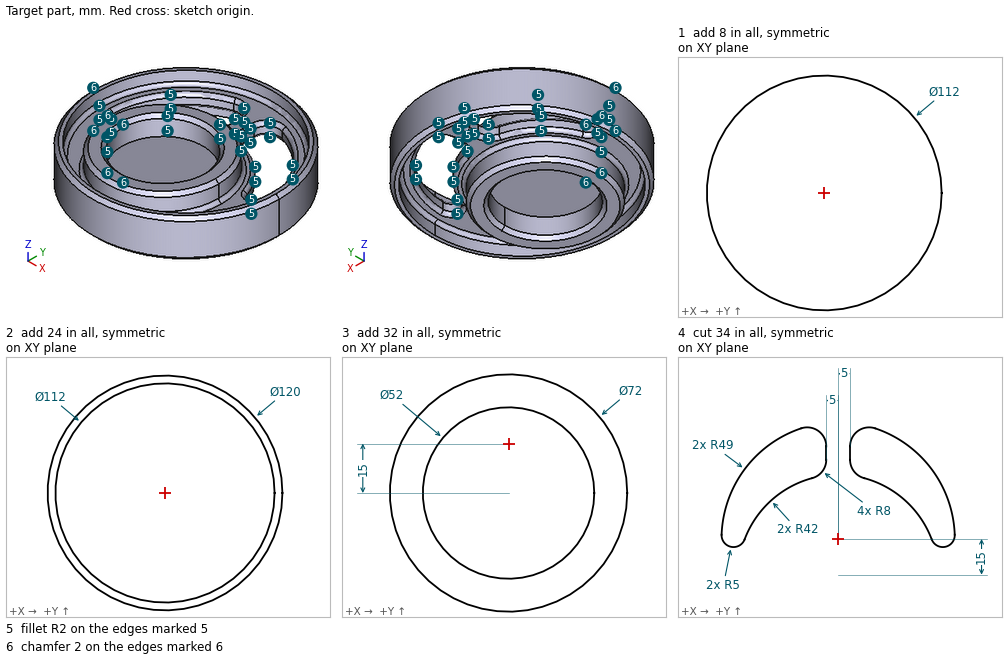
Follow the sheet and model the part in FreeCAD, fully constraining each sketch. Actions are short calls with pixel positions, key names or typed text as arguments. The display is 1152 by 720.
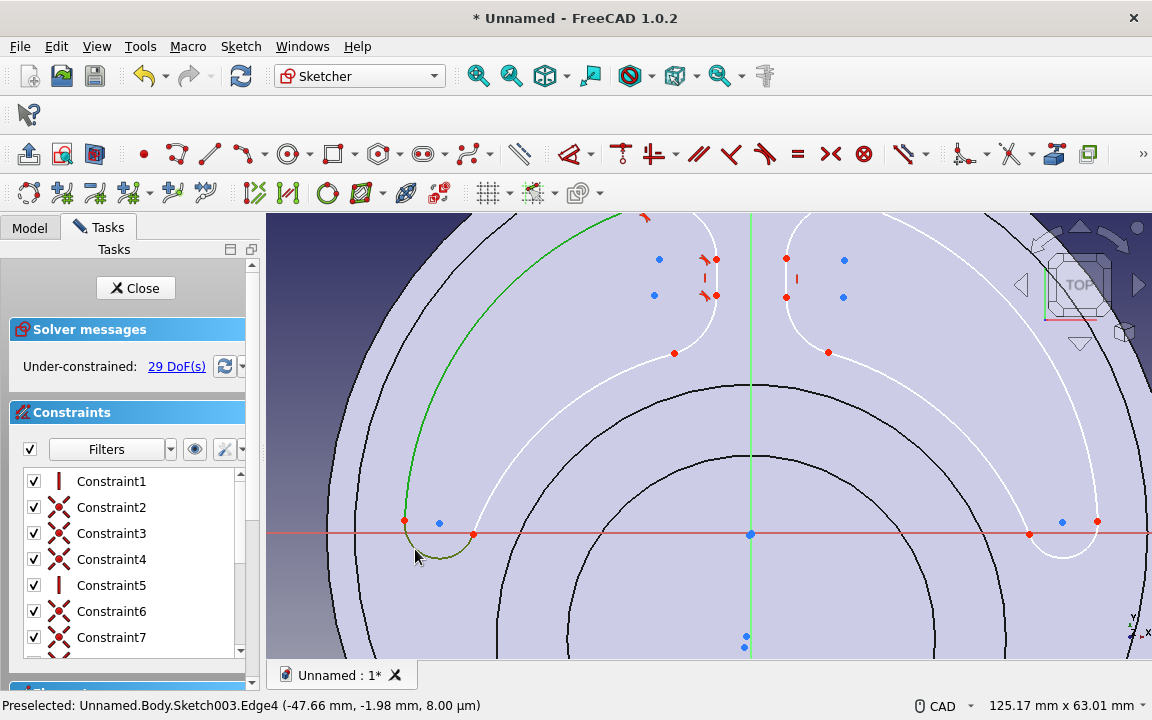
key(t)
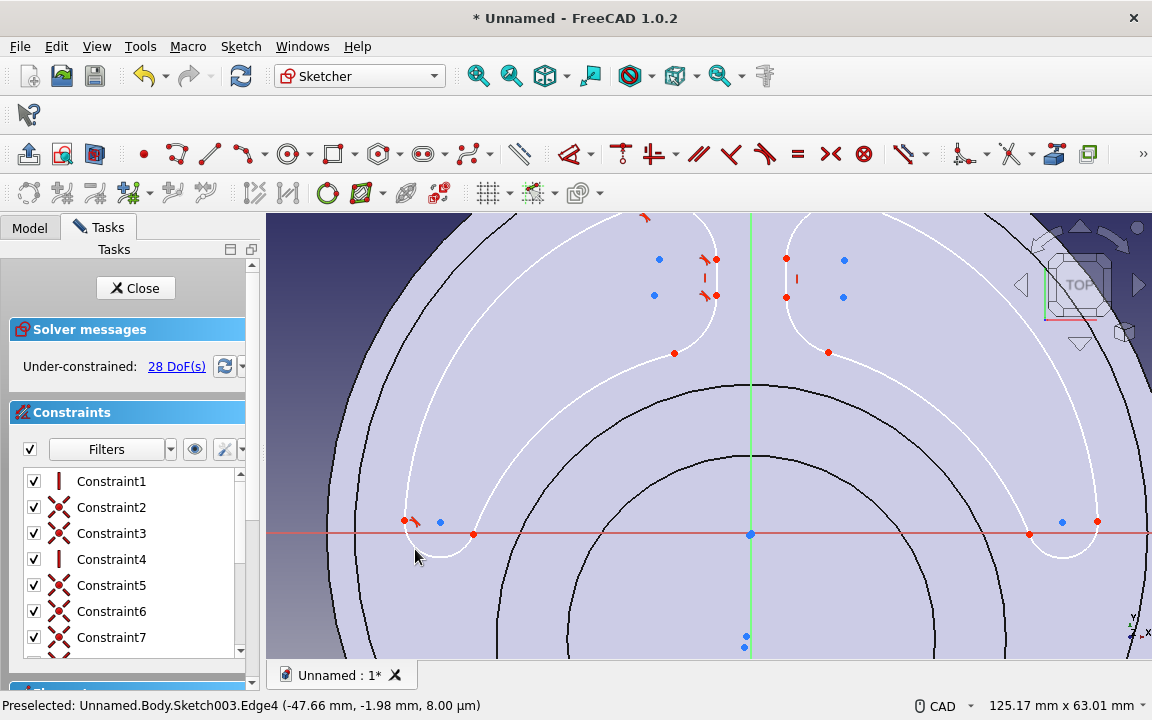
click(416, 548)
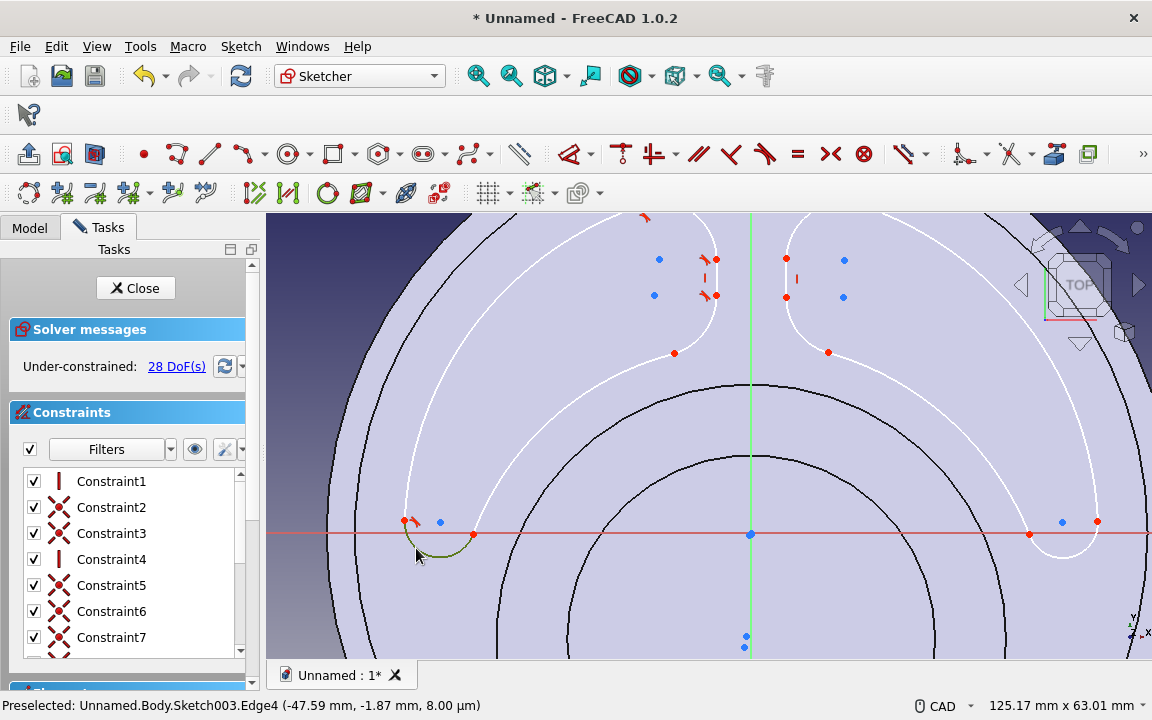
click(597, 386)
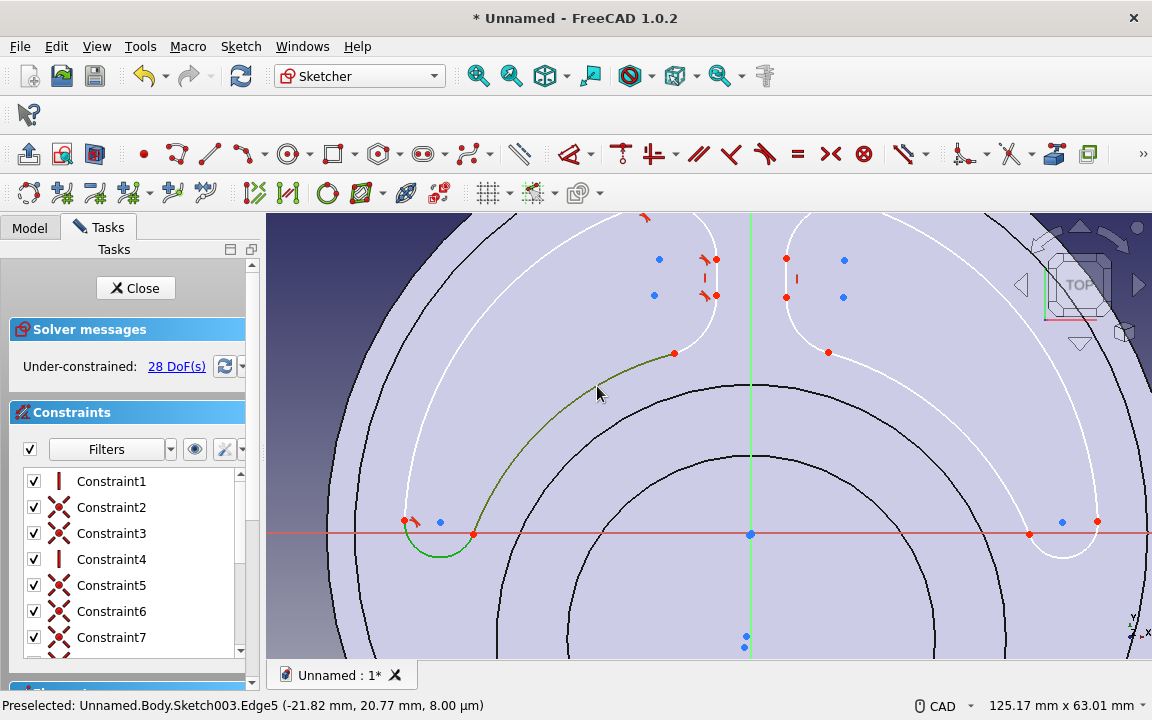
key(t)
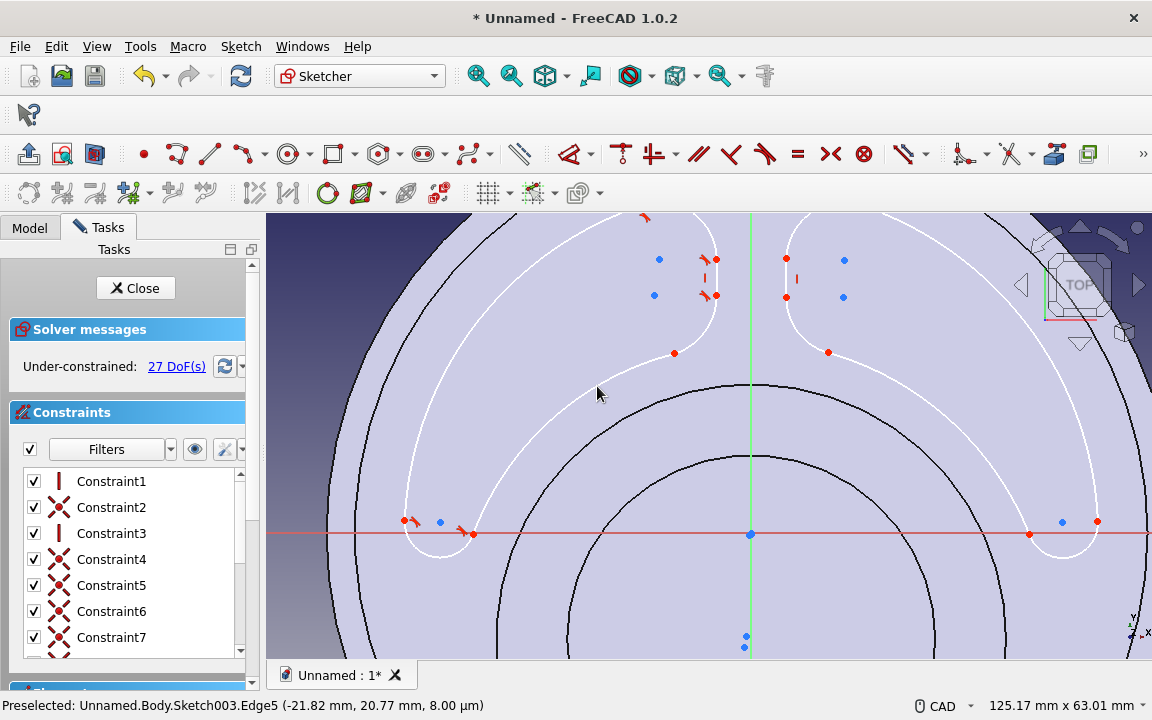
click(597, 386)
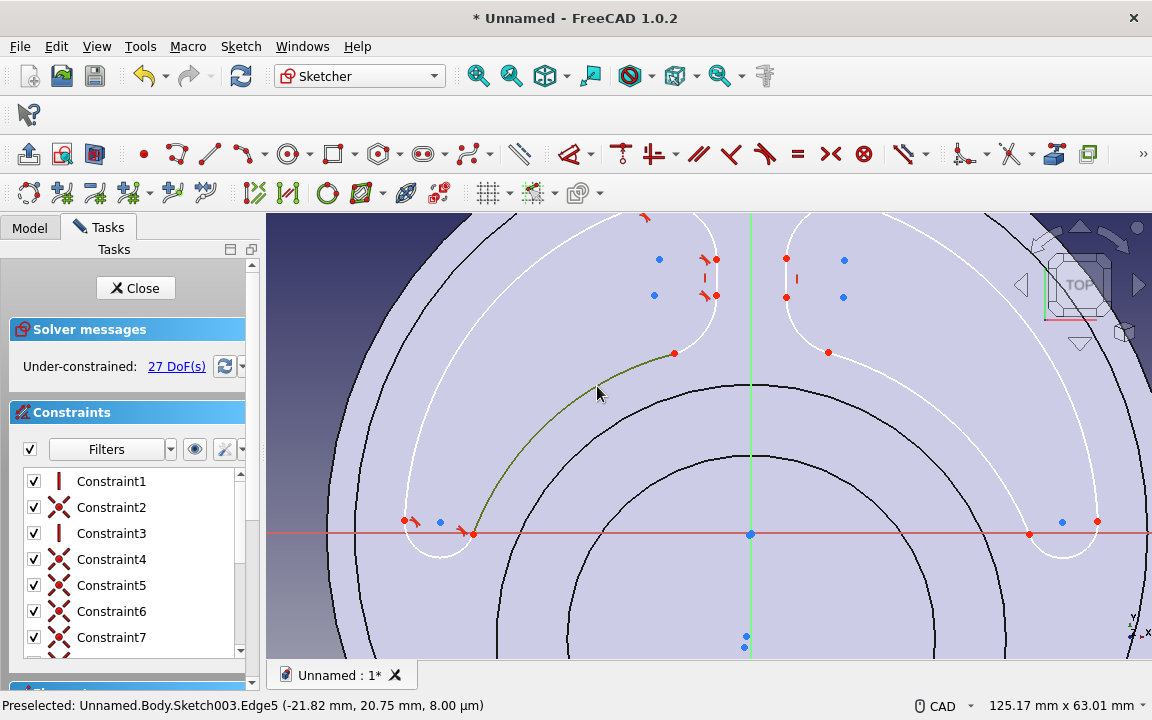
click(695, 343)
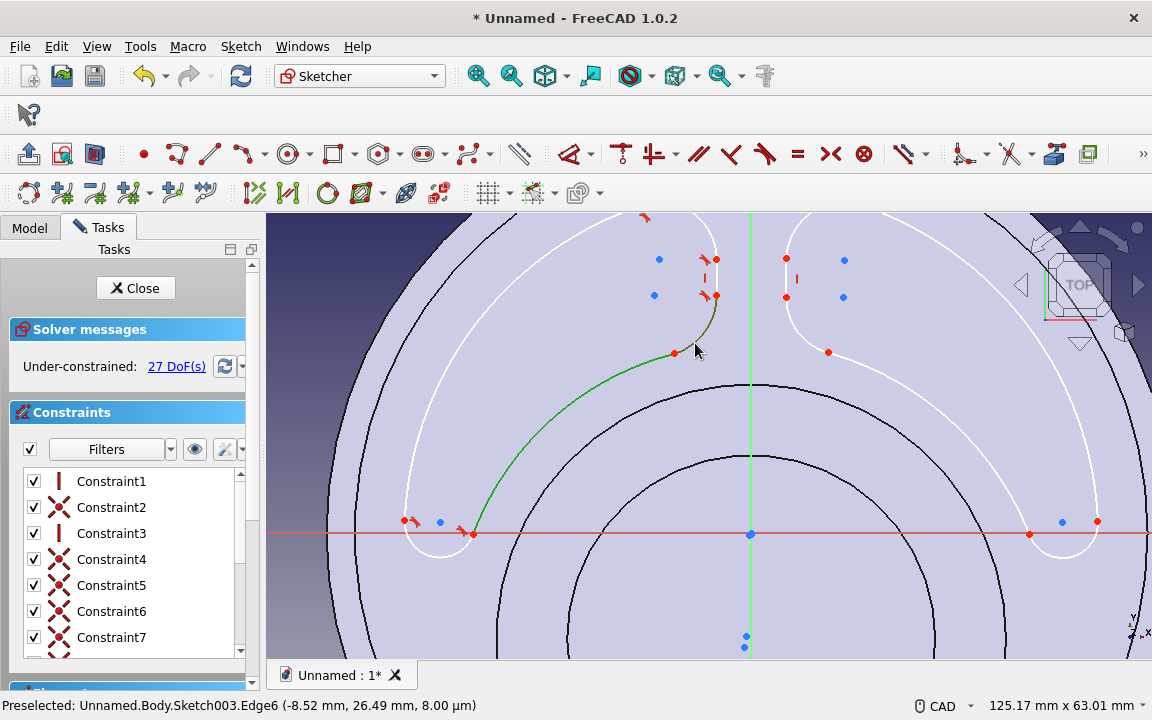
key(t)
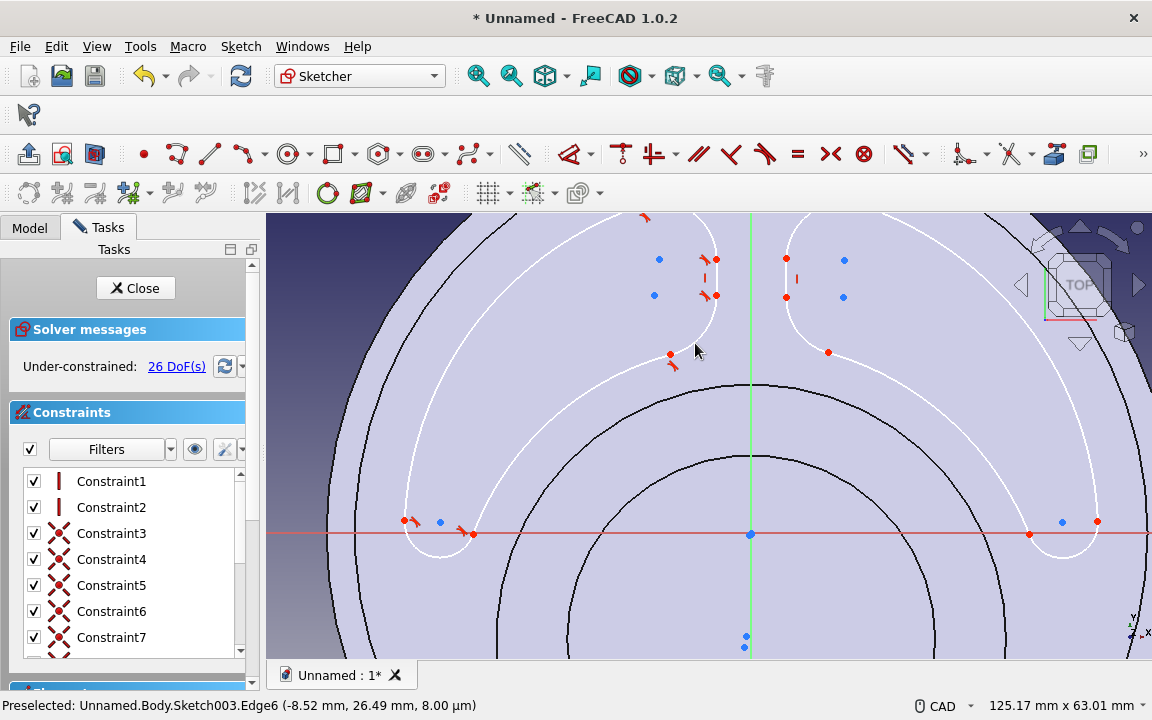
click(786, 270)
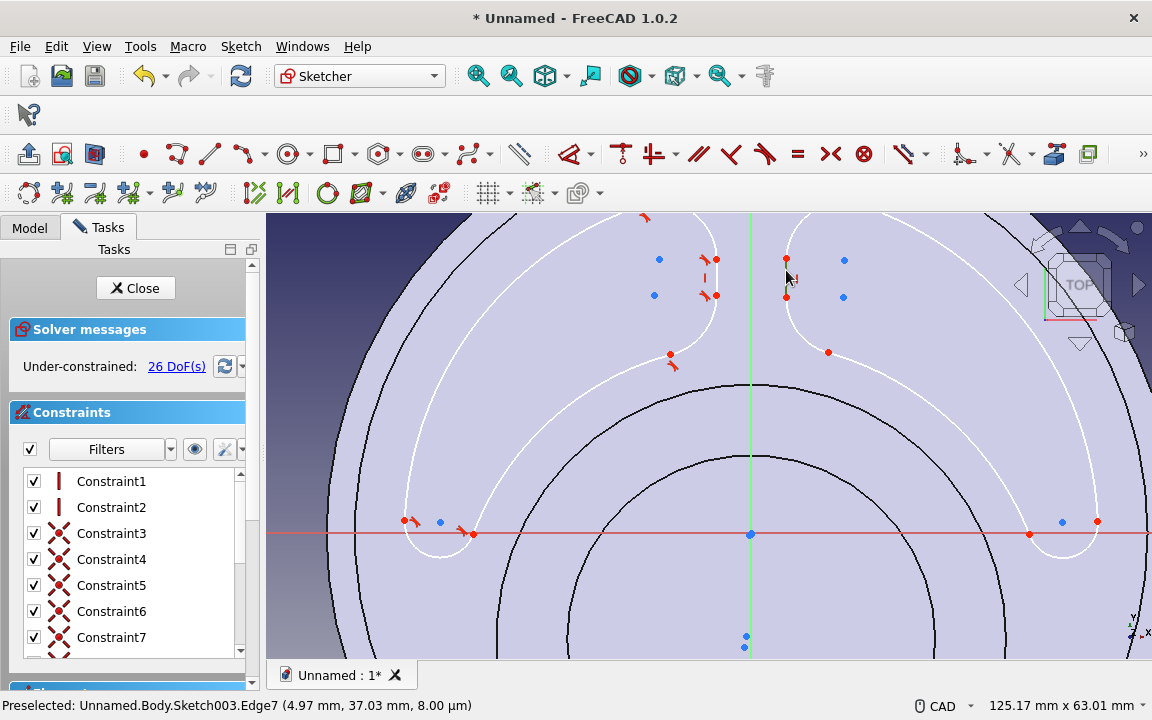
click(791, 320)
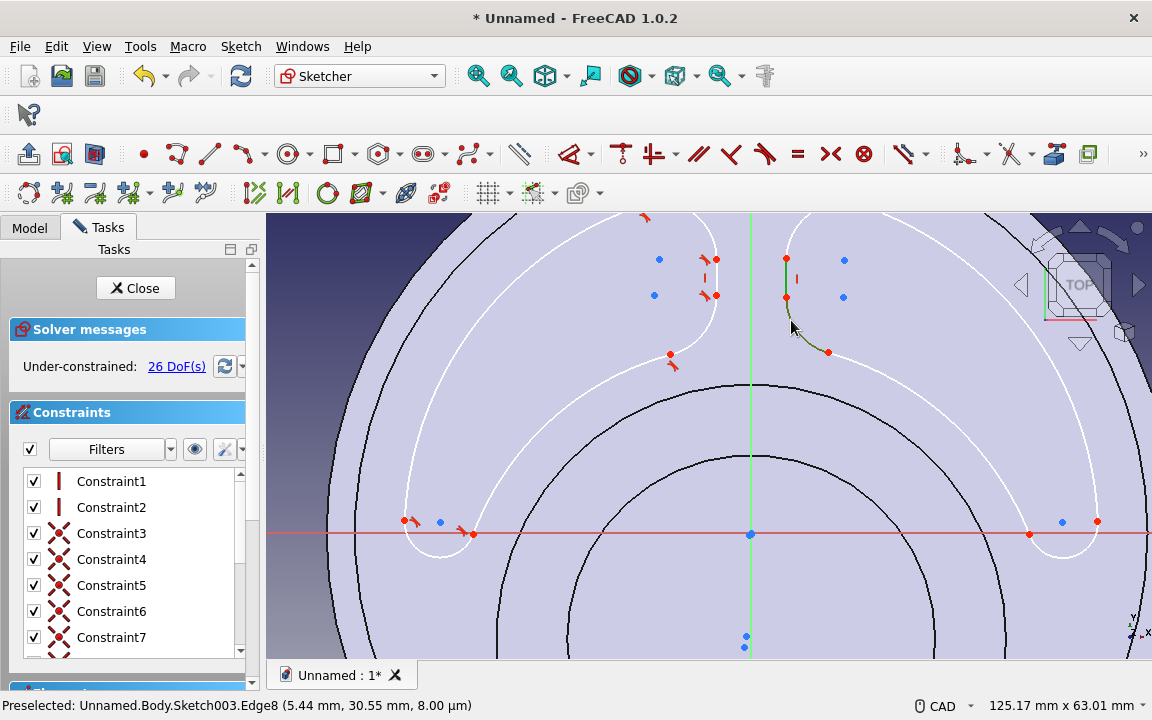
key(t)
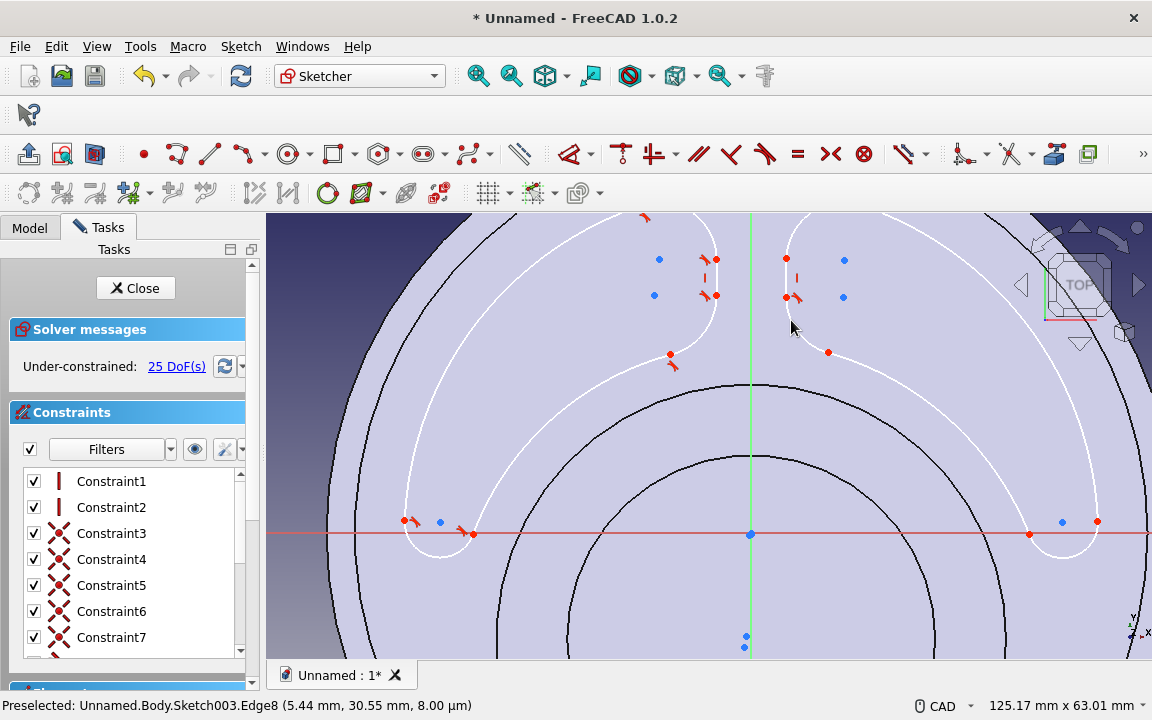
click(786, 270)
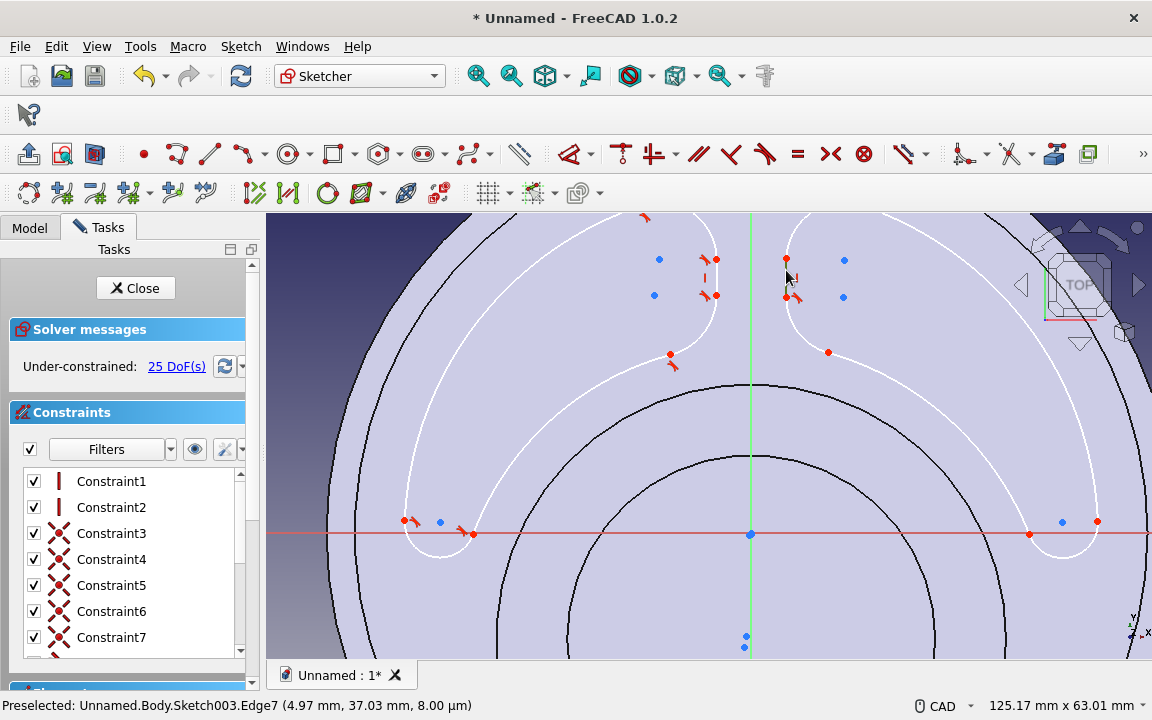
scroll(415, 549, down, 2)